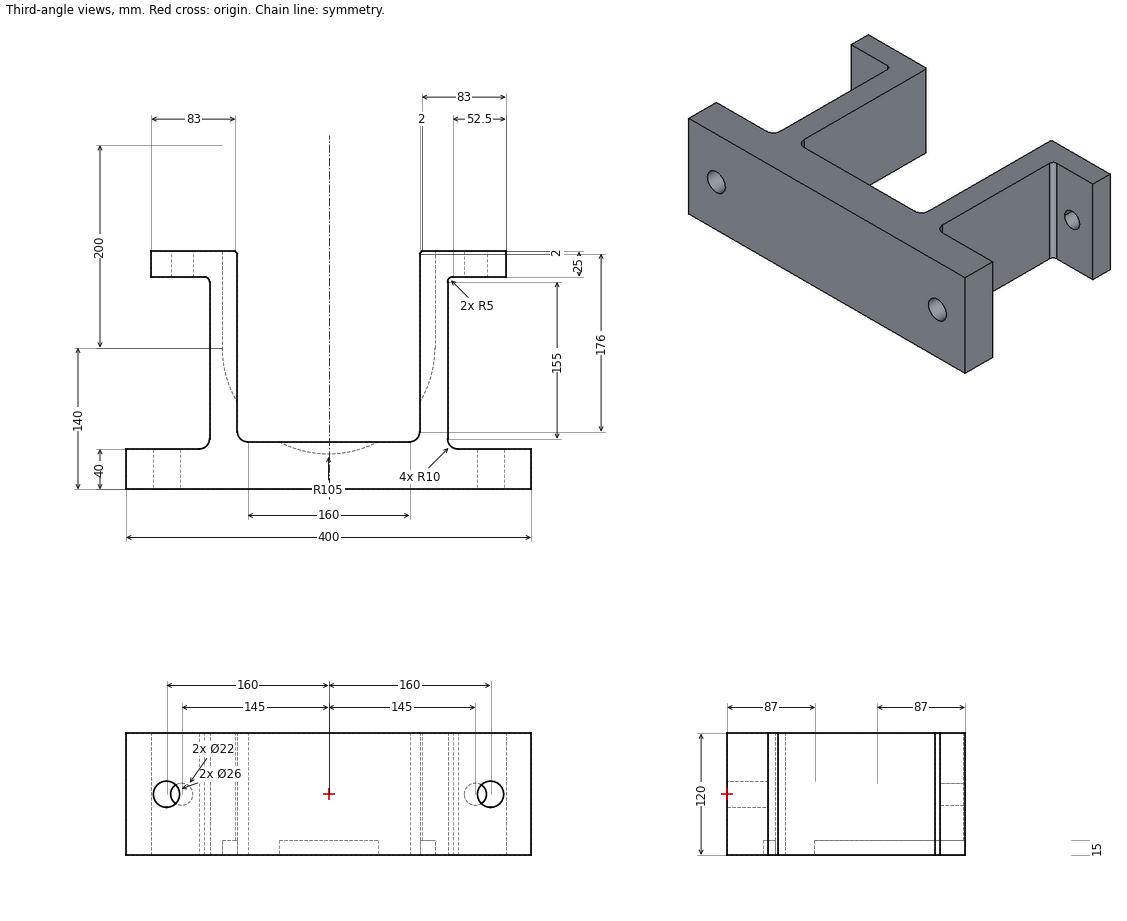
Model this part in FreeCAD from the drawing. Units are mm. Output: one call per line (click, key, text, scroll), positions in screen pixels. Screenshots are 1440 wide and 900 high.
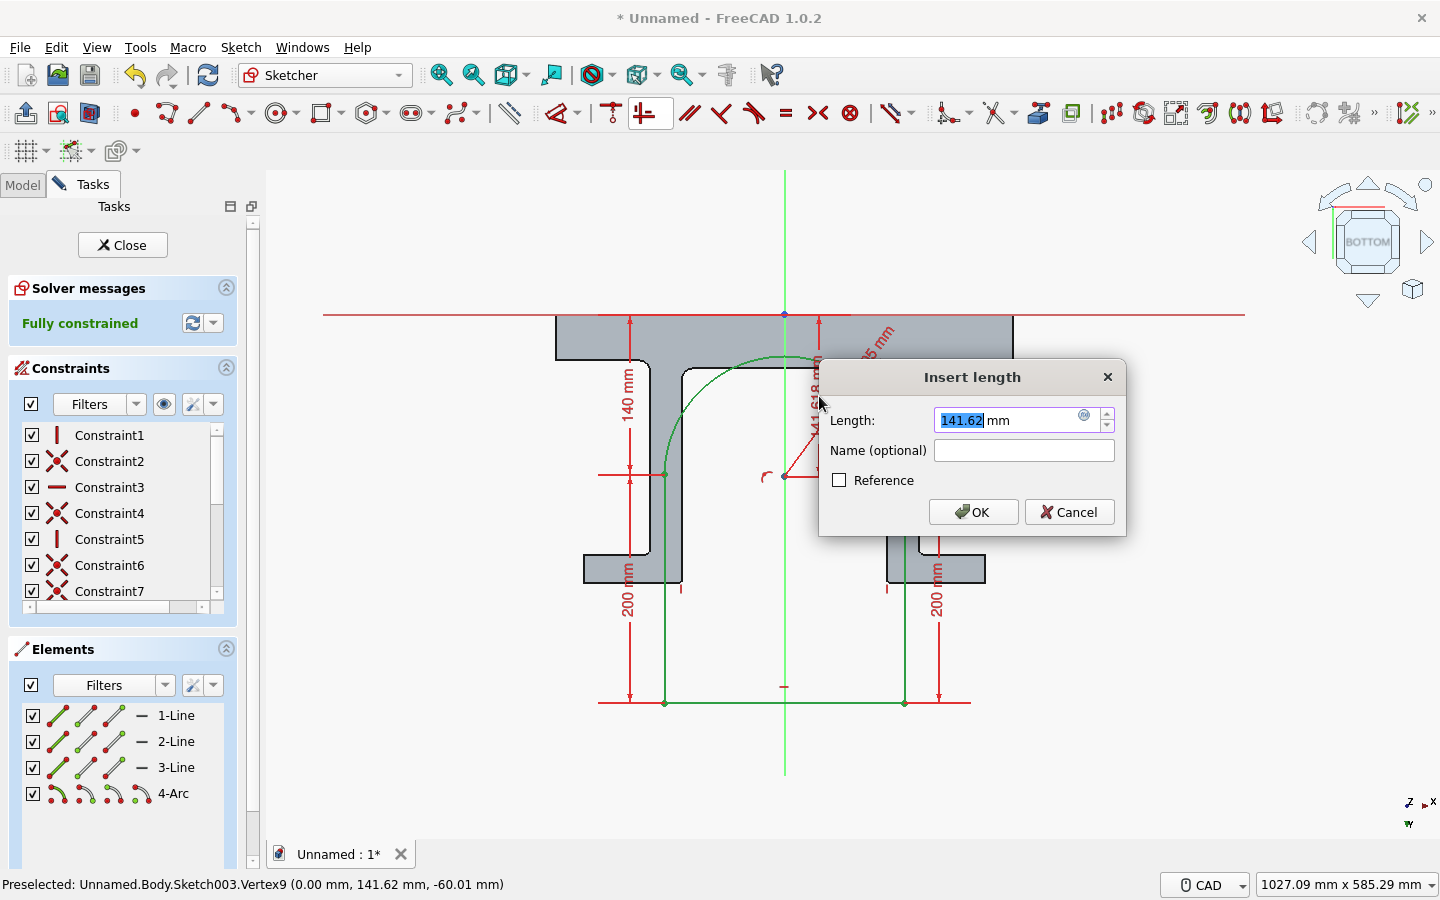
text(140)
key(Return)
key(Escape)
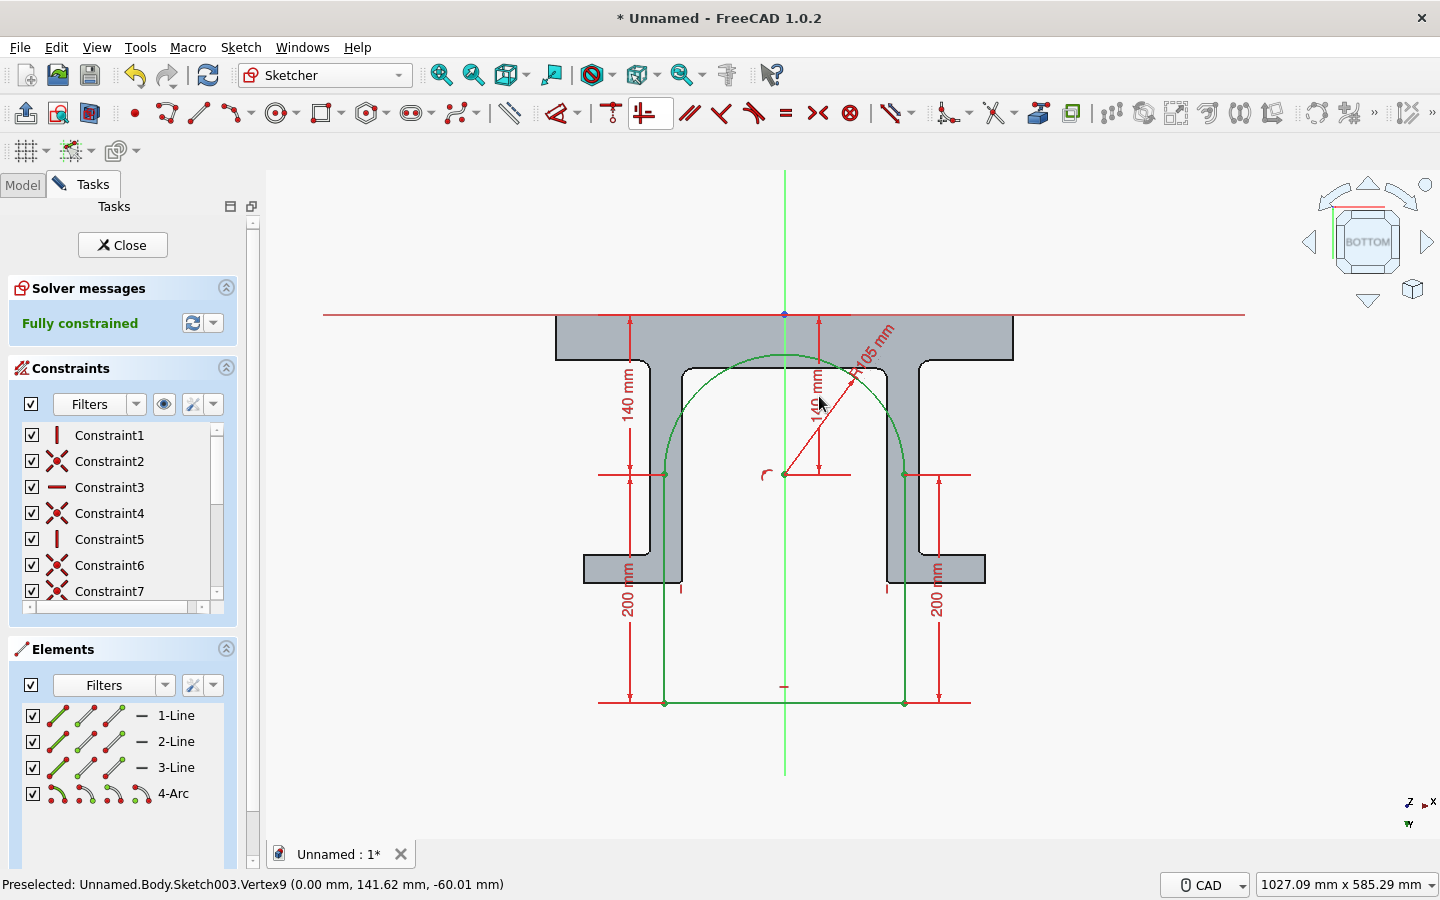
click(123, 245)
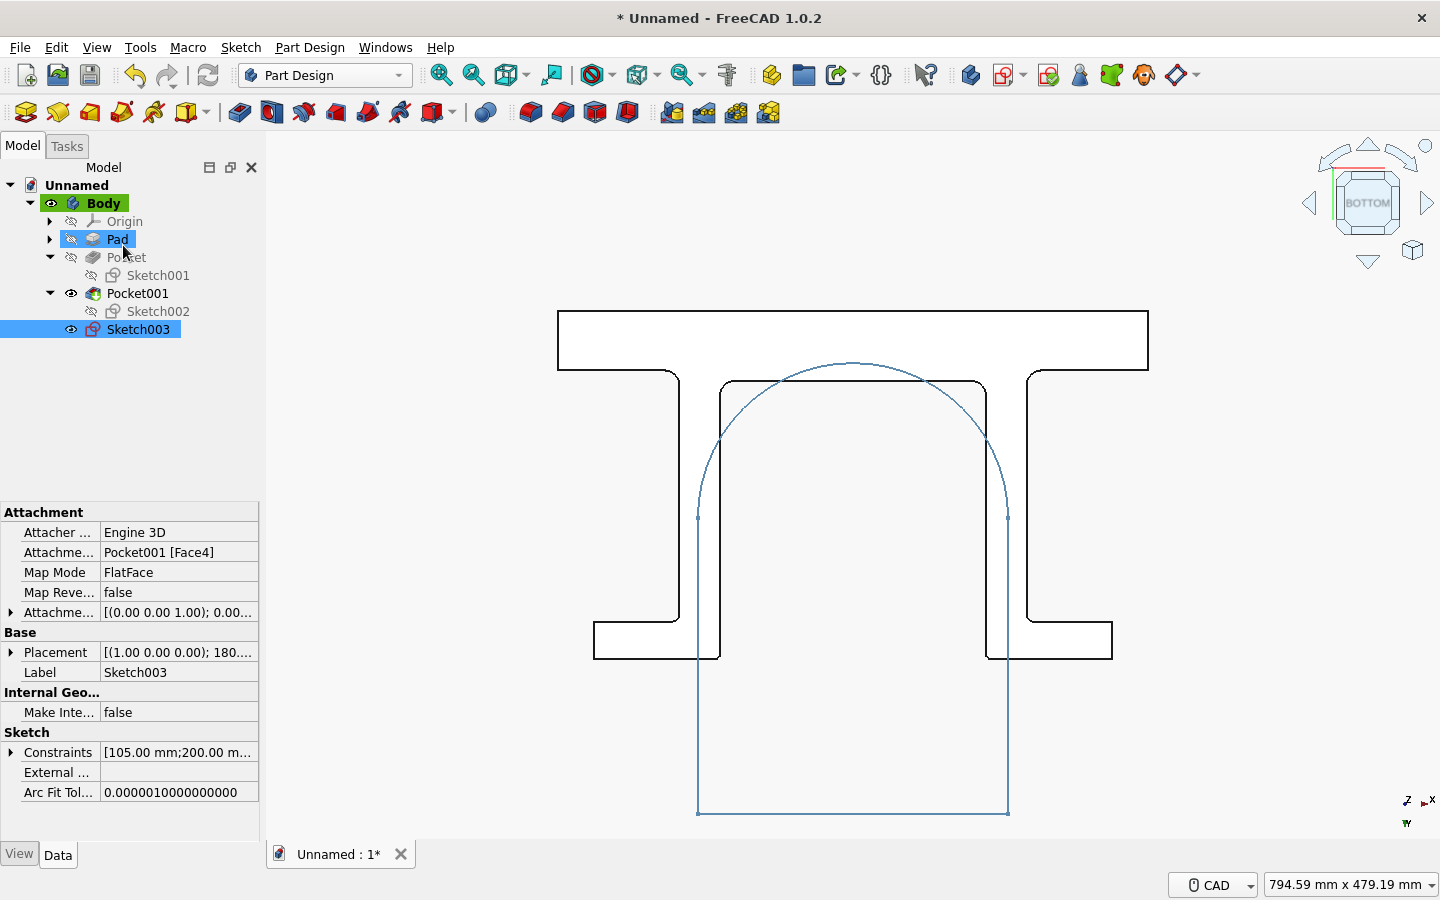
click(240, 112)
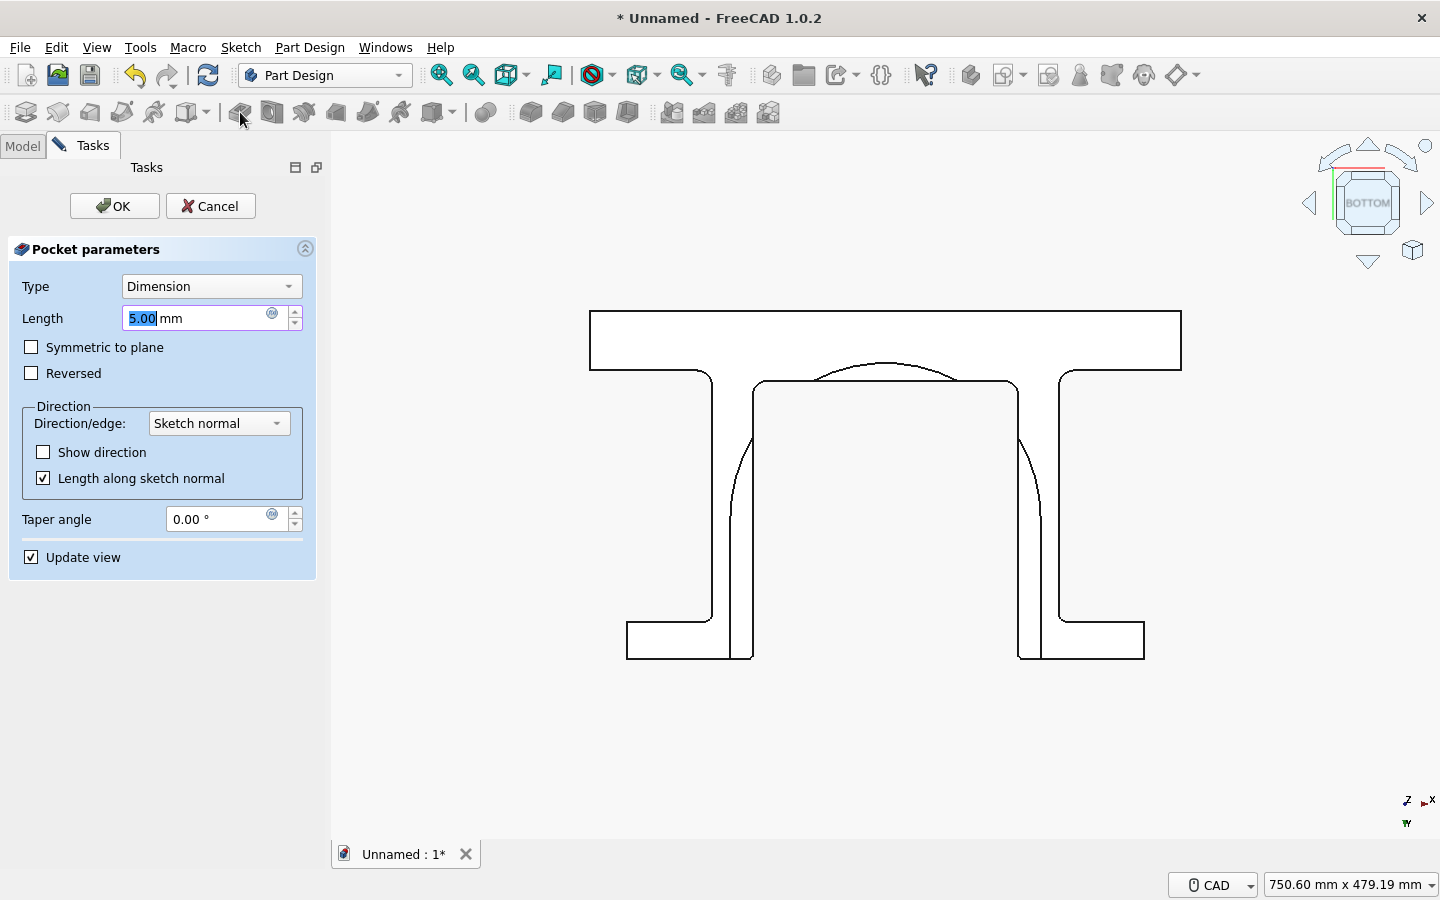
text(15)
key(Tab)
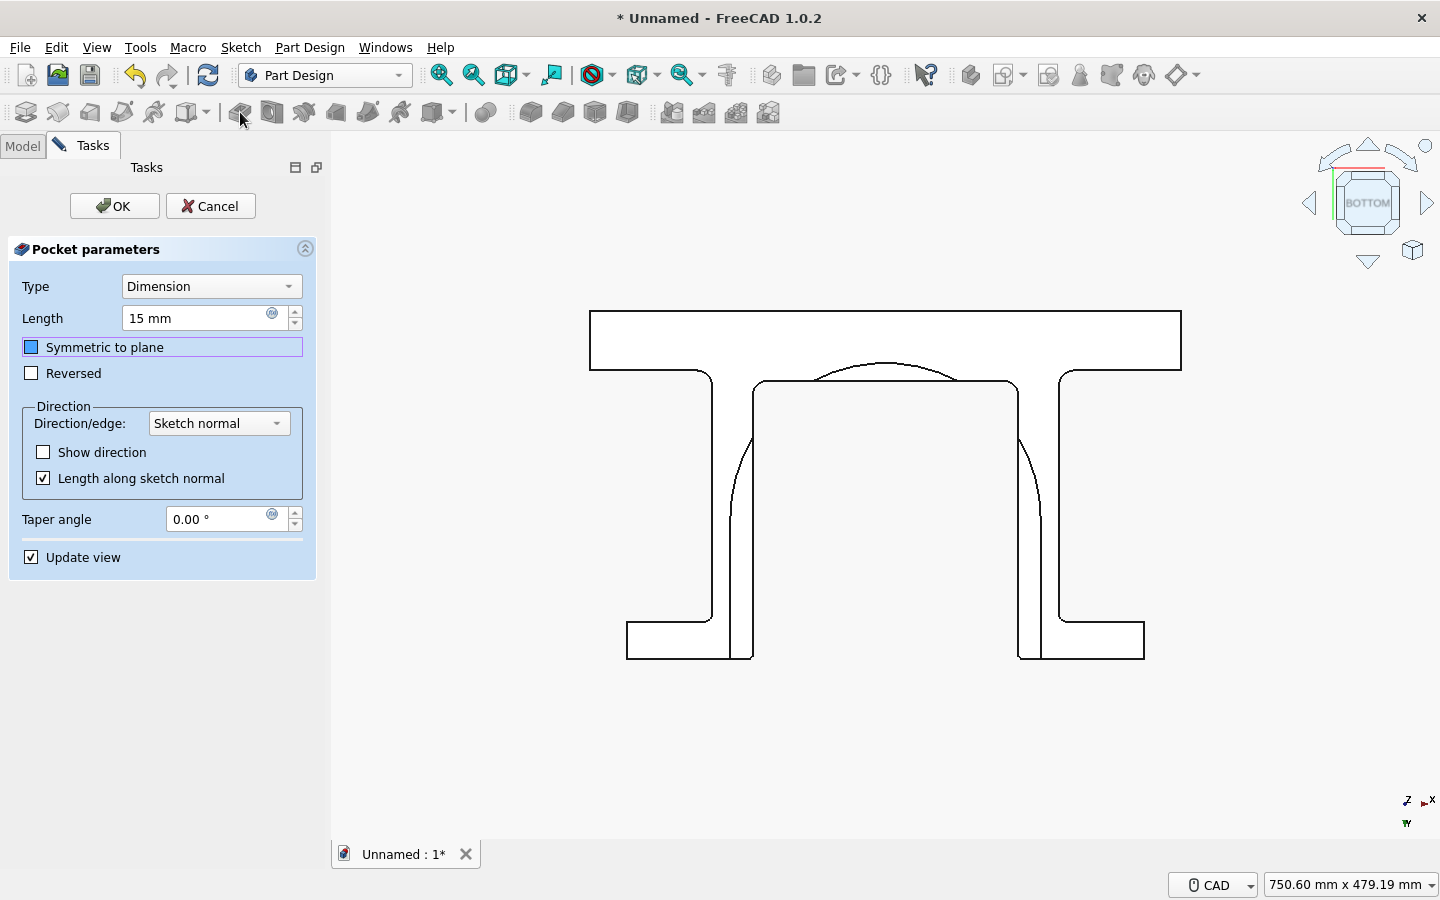
click(115, 206)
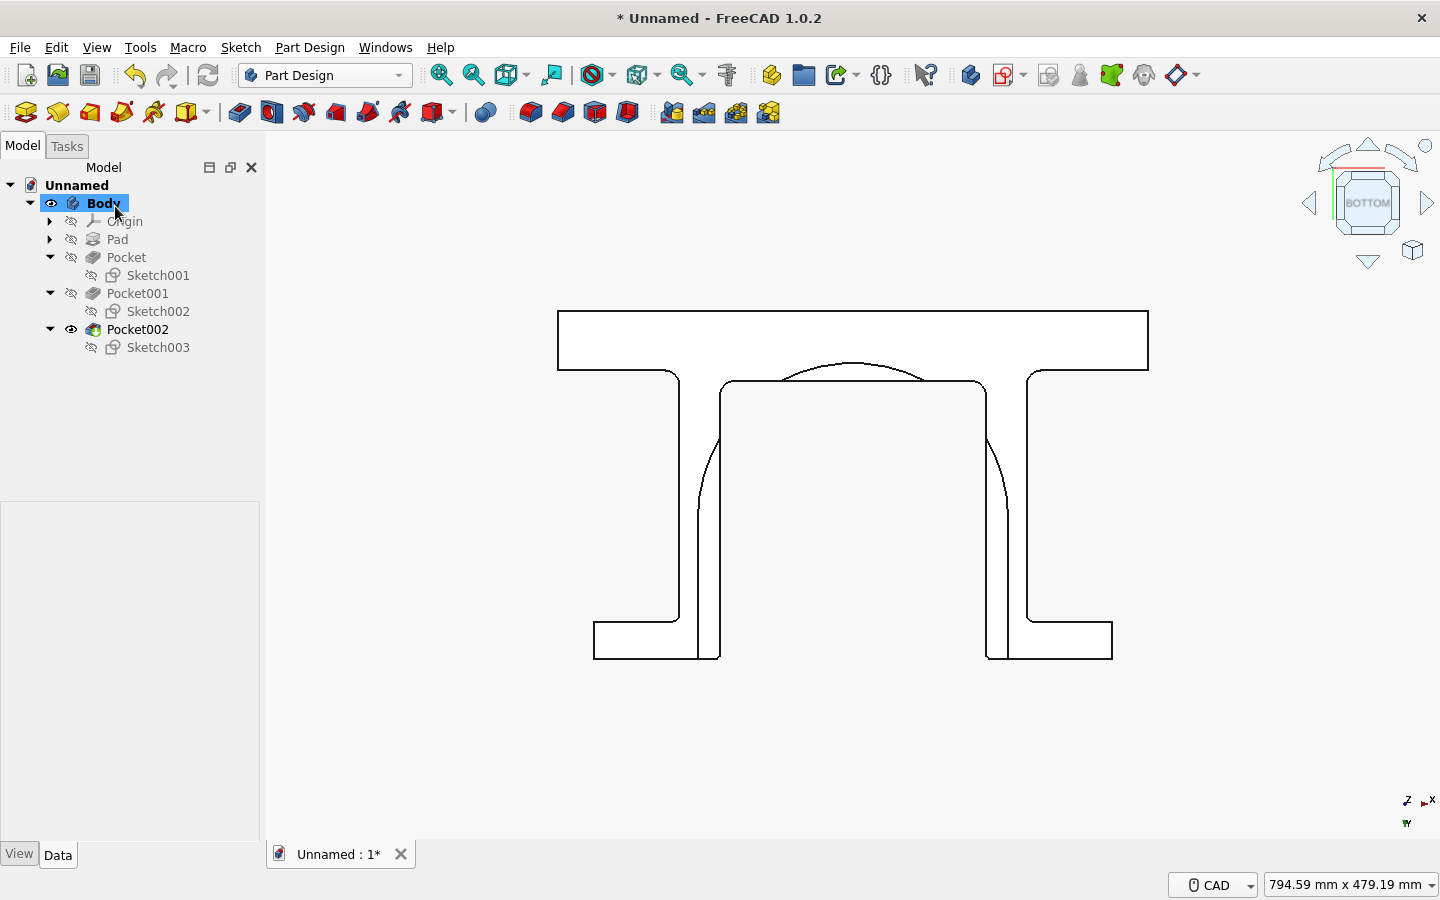
key(0)